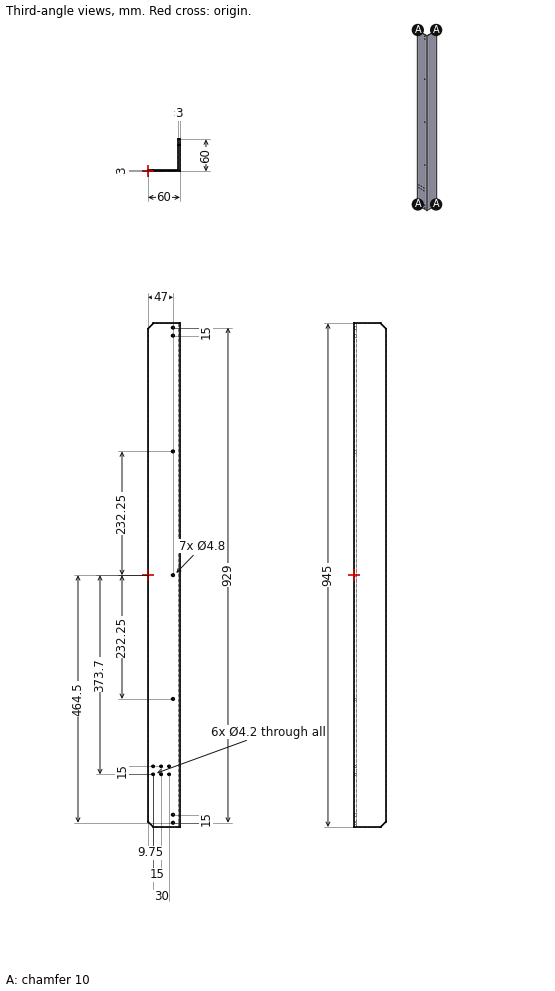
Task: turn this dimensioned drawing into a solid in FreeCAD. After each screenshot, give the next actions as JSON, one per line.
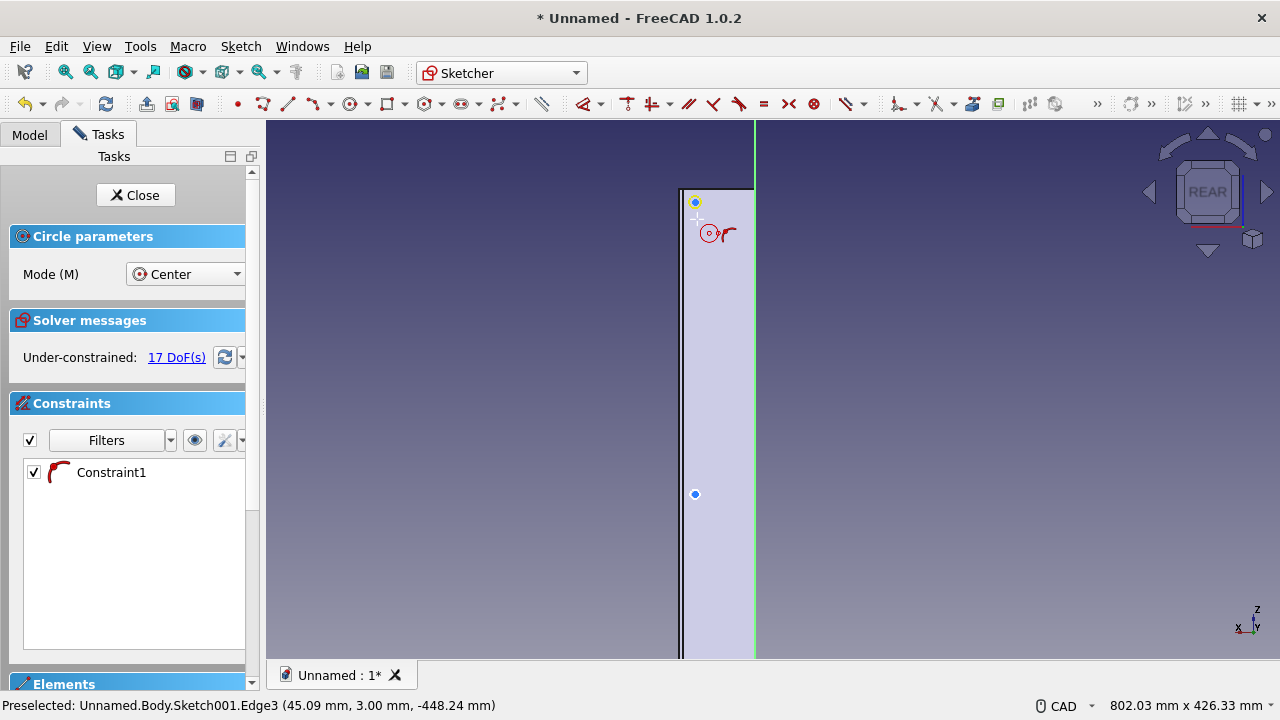
{"action": "left_click", "coordinate": [695, 218]}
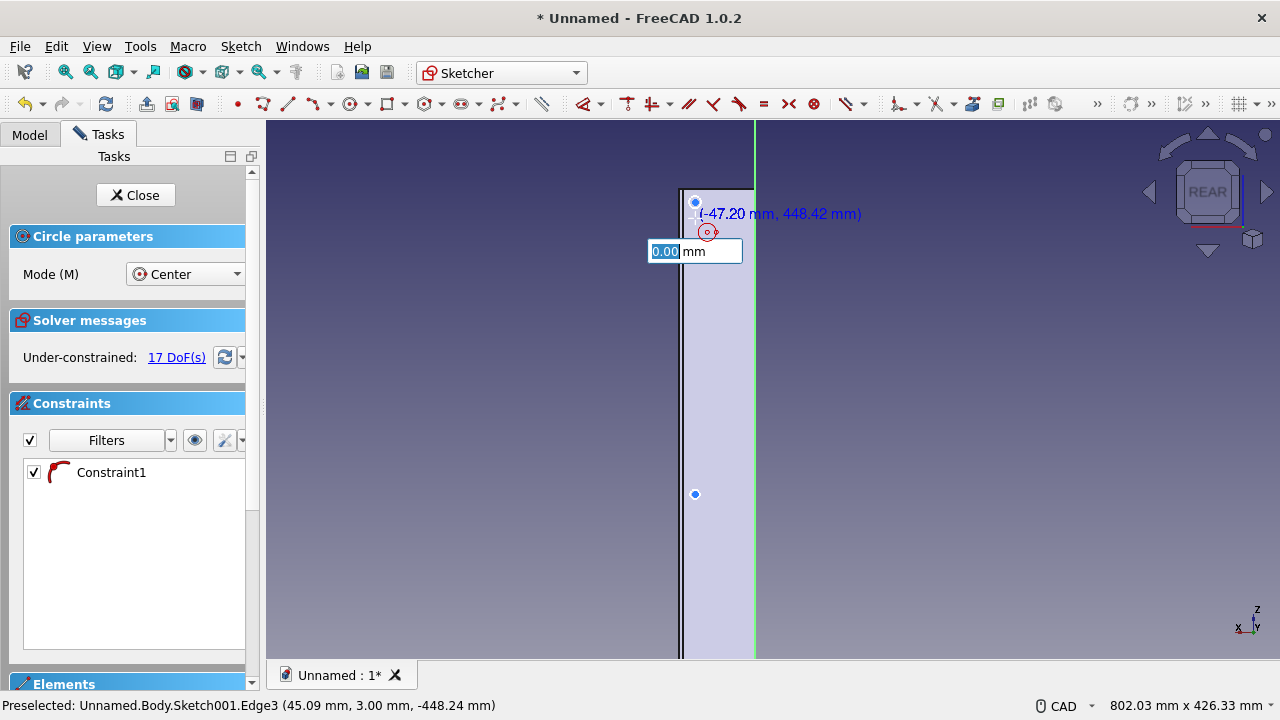
{"action": "scroll", "coordinate": [697, 220], "scroll_direction": "up", "scroll_amount": 9}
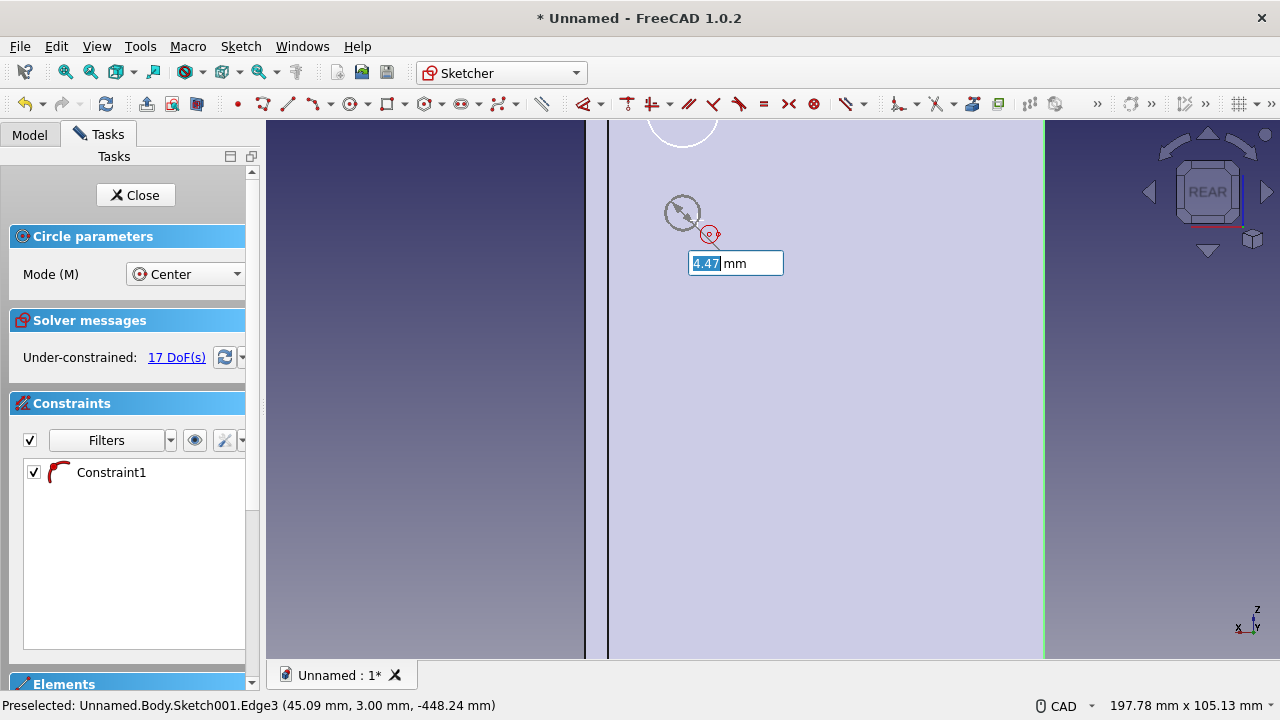
{"action": "left_click", "coordinate": [697, 218]}
{"action": "key", "text": "Escape"}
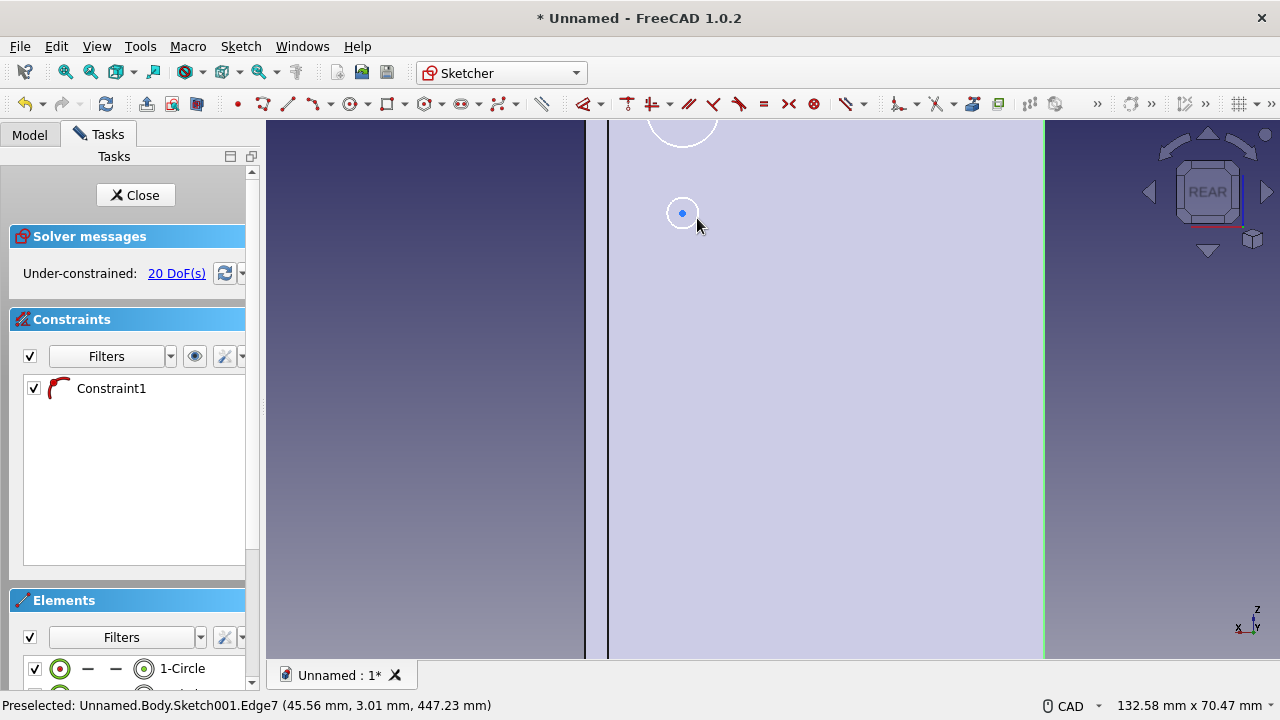
{"action": "scroll", "coordinate": [697, 219], "scroll_direction": "down", "scroll_amount": 15}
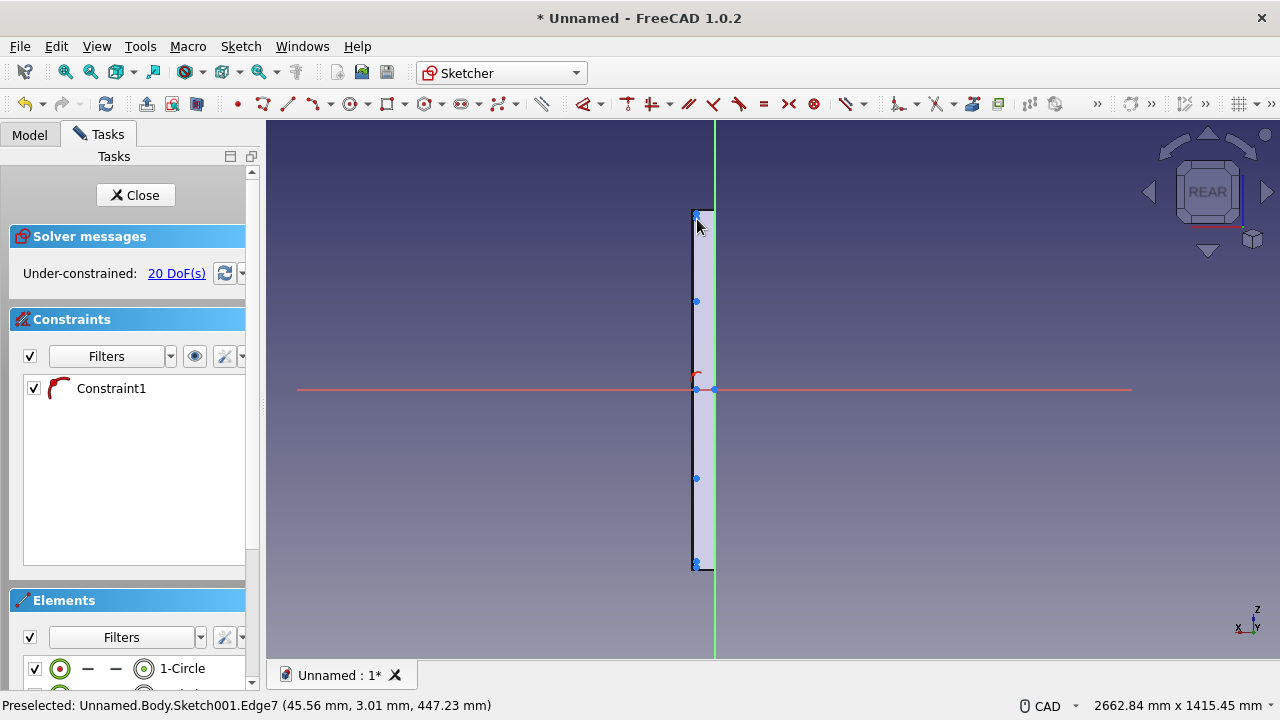
{"action": "scroll", "coordinate": [697, 389], "scroll_direction": "up", "scroll_amount": 14}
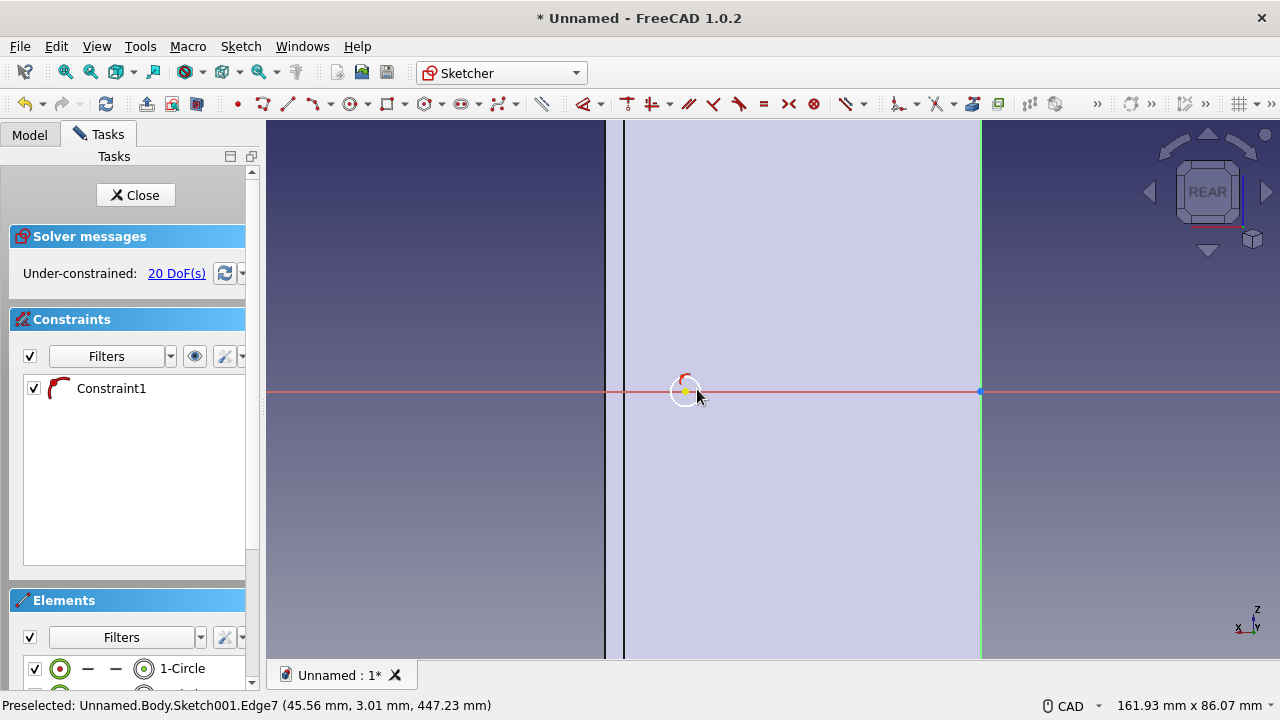
{"action": "left_click", "coordinate": [696, 381]}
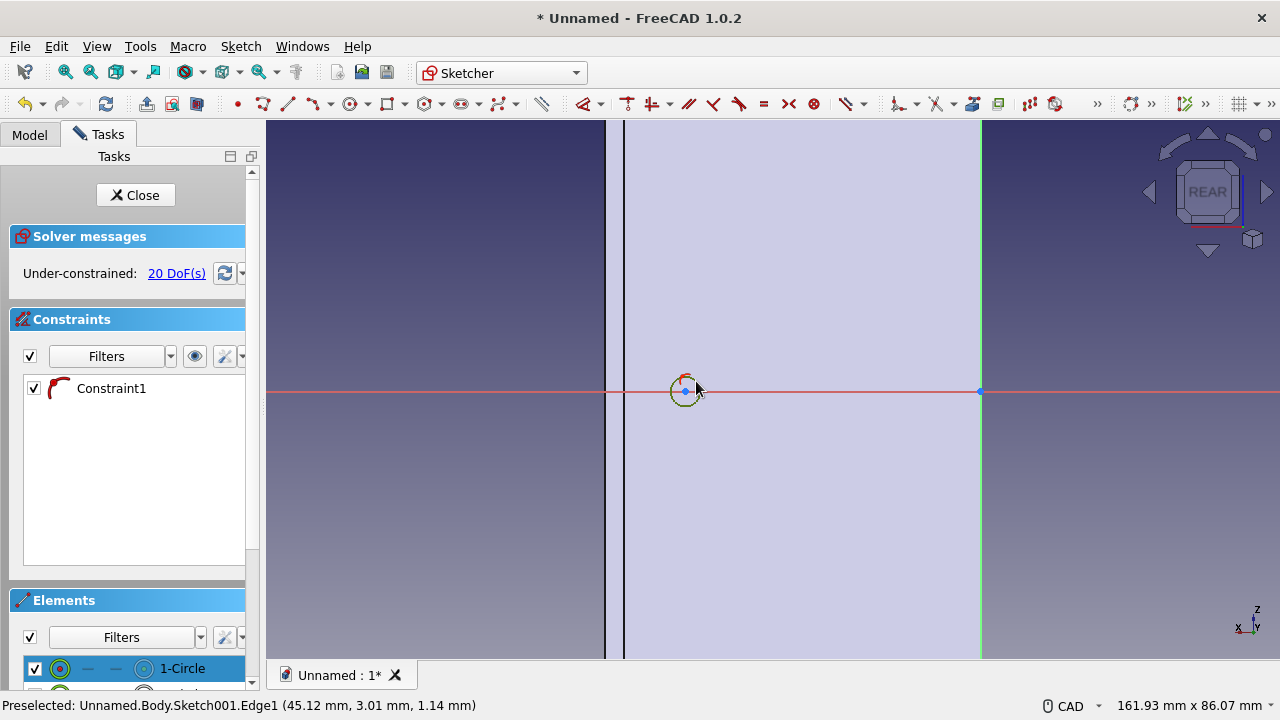
{"action": "scroll", "coordinate": [697, 389], "scroll_direction": "down", "scroll_amount": 14}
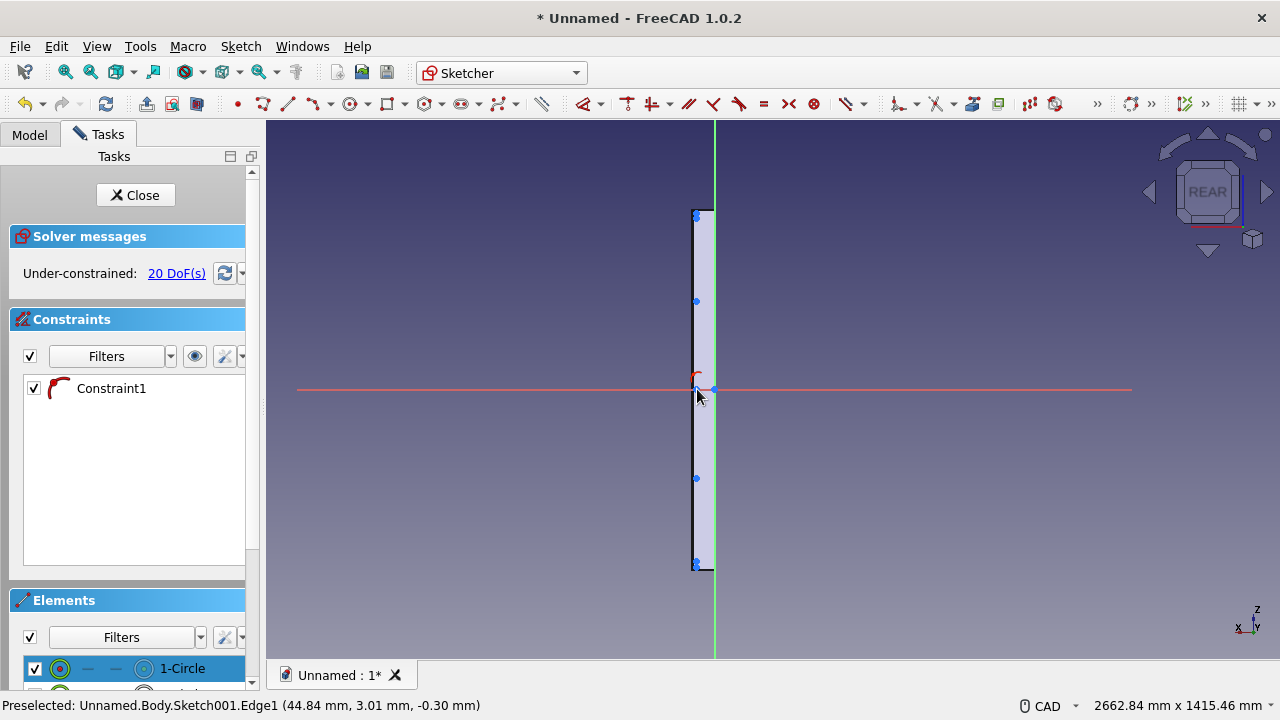
{"action": "scroll", "coordinate": [698, 478], "scroll_direction": "up", "scroll_amount": 12}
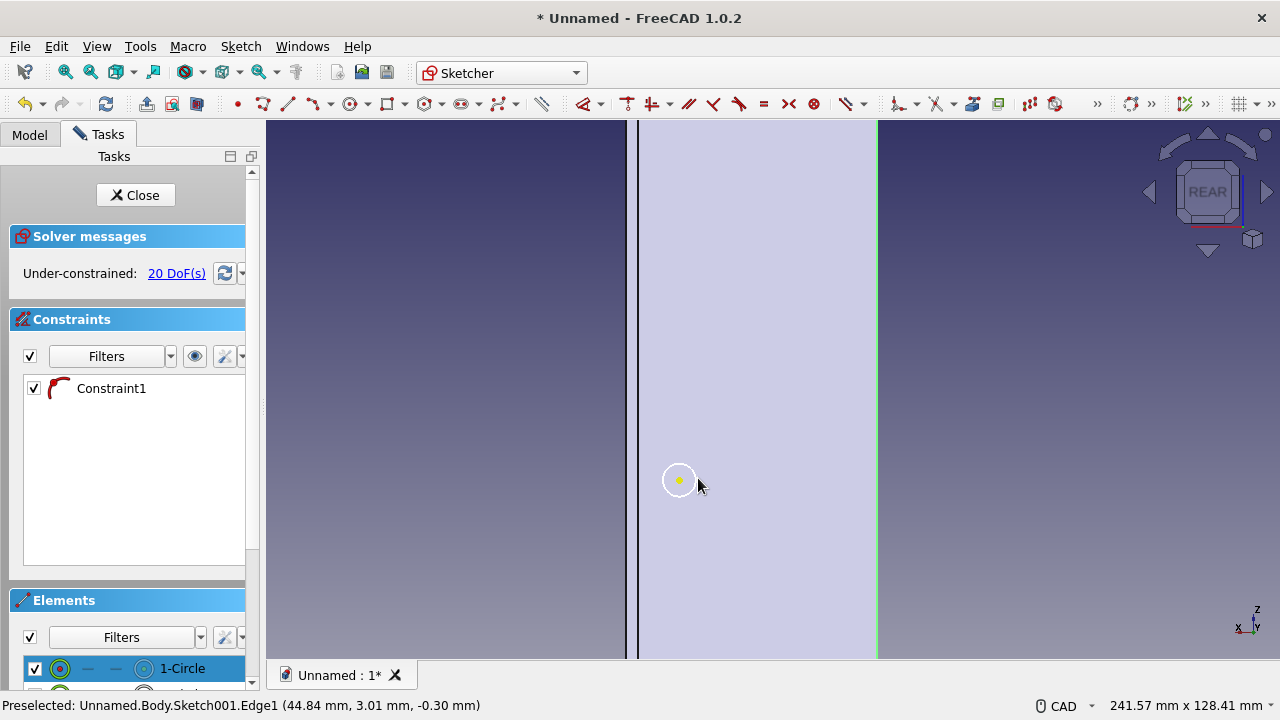
{"action": "left_click", "coordinate": [691, 469]}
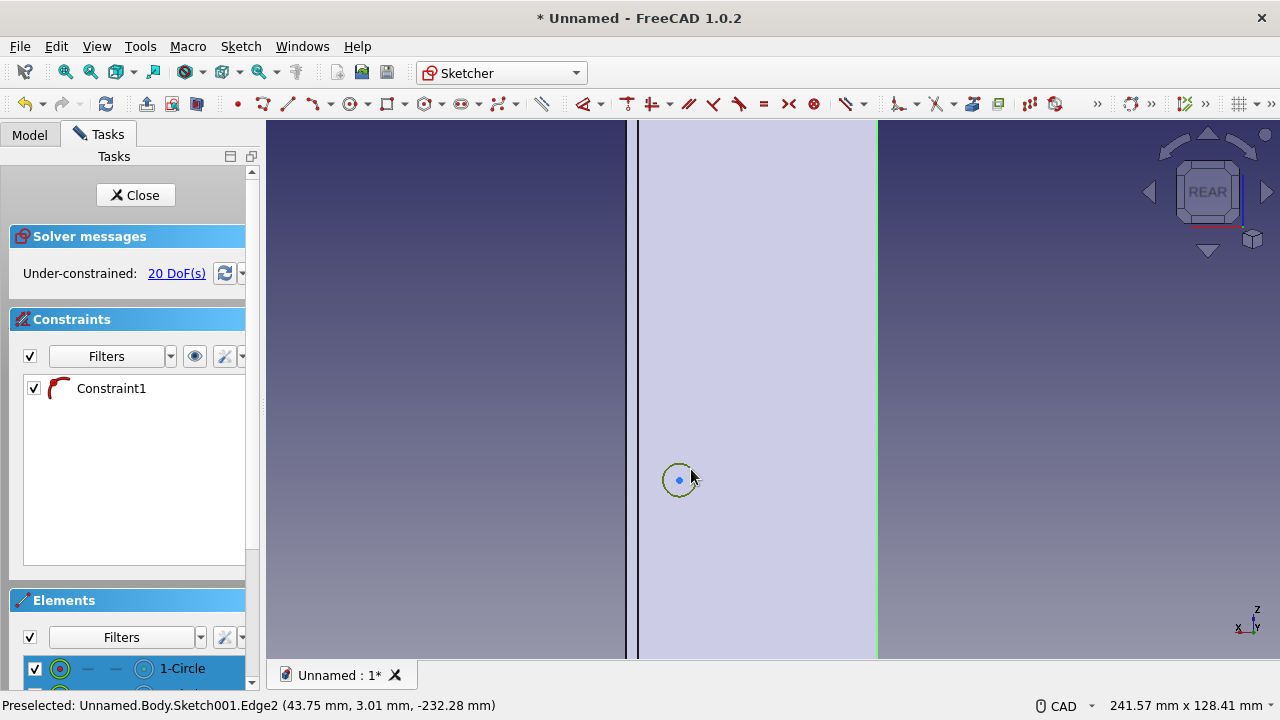
{"action": "scroll", "coordinate": [698, 479], "scroll_direction": "down", "scroll_amount": 12}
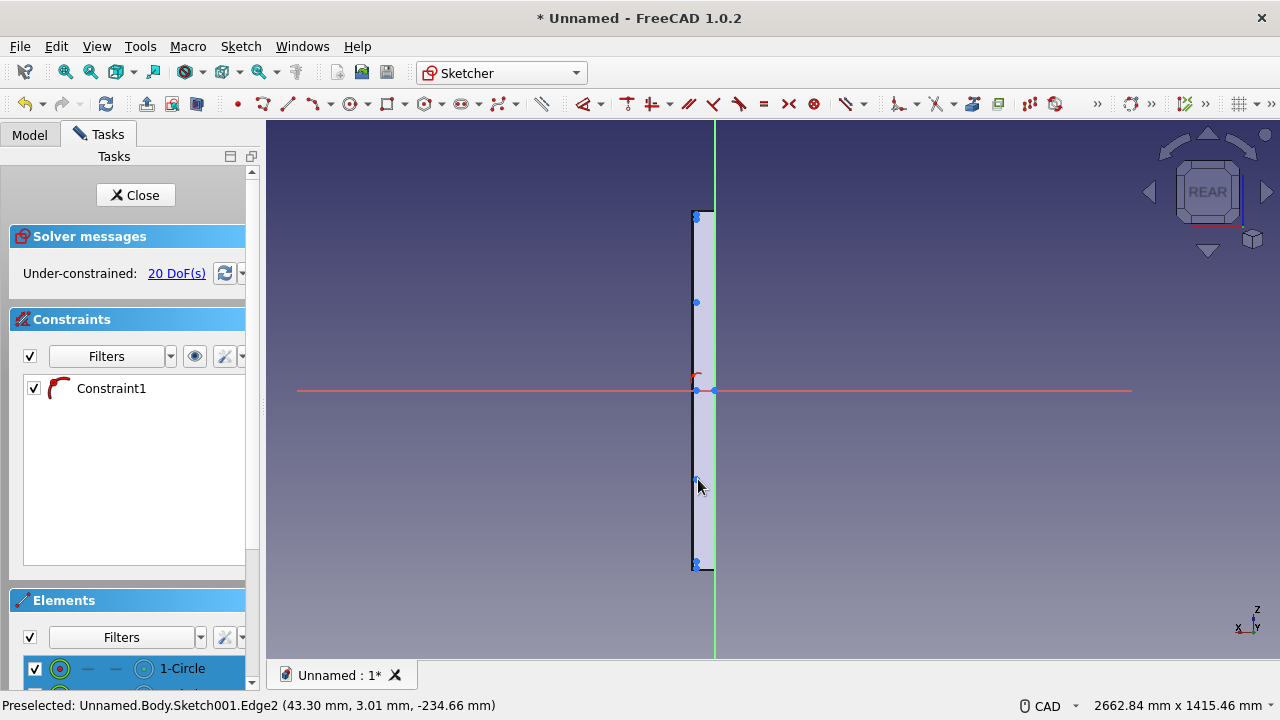
{"action": "scroll", "coordinate": [698, 567], "scroll_direction": "up", "scroll_amount": 10}